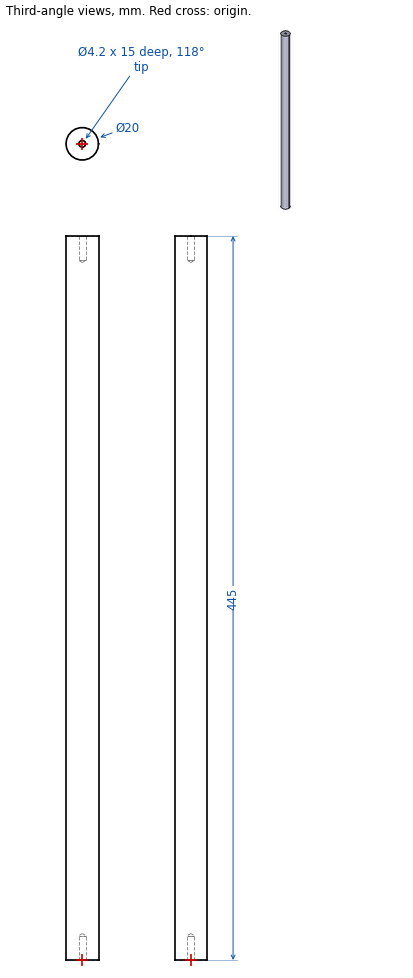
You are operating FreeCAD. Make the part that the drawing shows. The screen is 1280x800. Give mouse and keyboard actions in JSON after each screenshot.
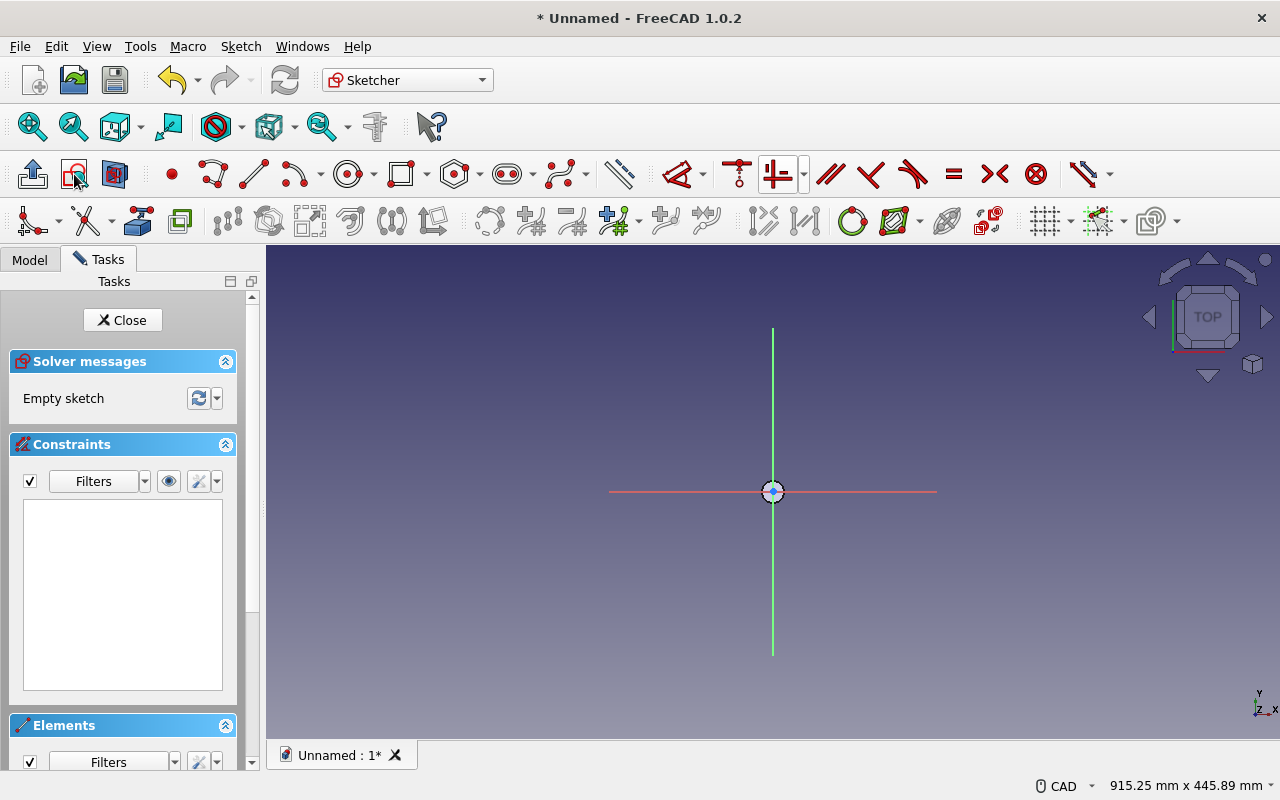
{"action": "scroll", "coordinate": [777, 492], "scroll_direction": "up", "scroll_amount": 15}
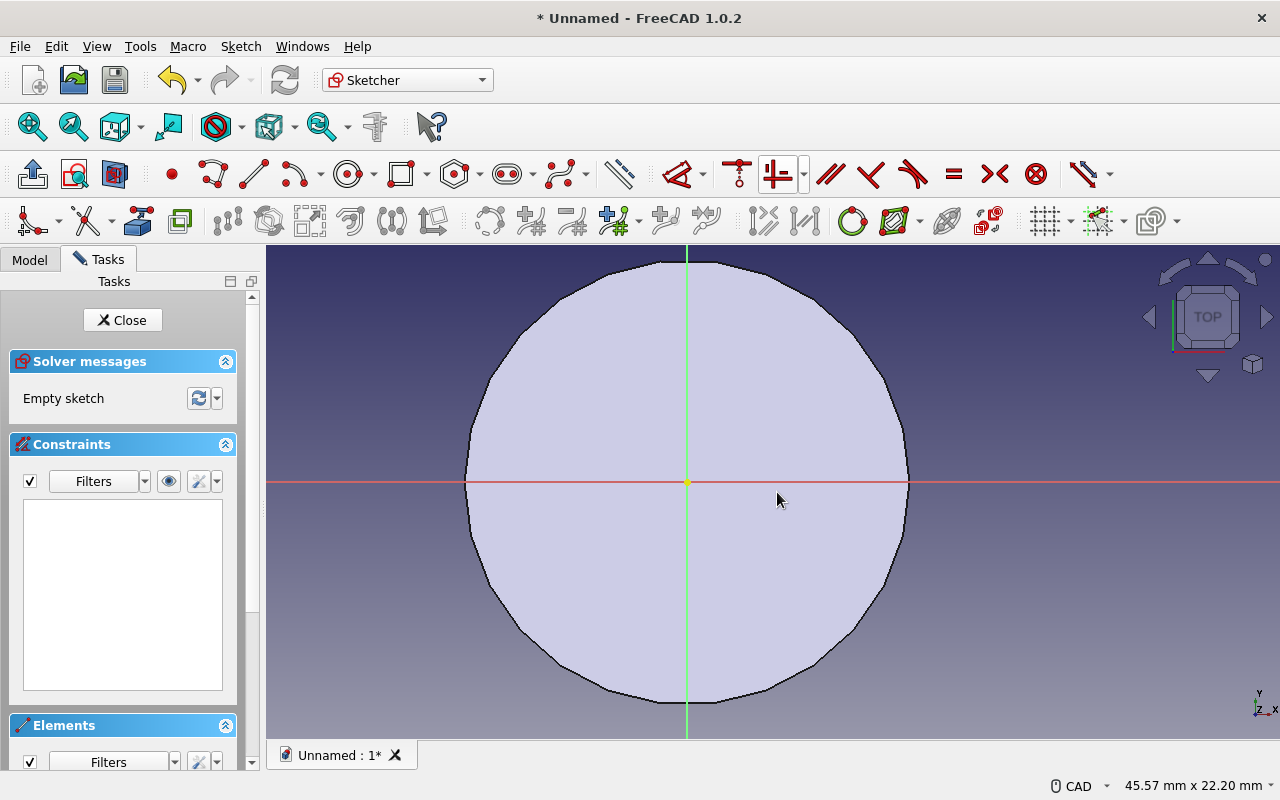
{"action": "scroll", "coordinate": [680, 478], "scroll_direction": "up", "scroll_amount": 6}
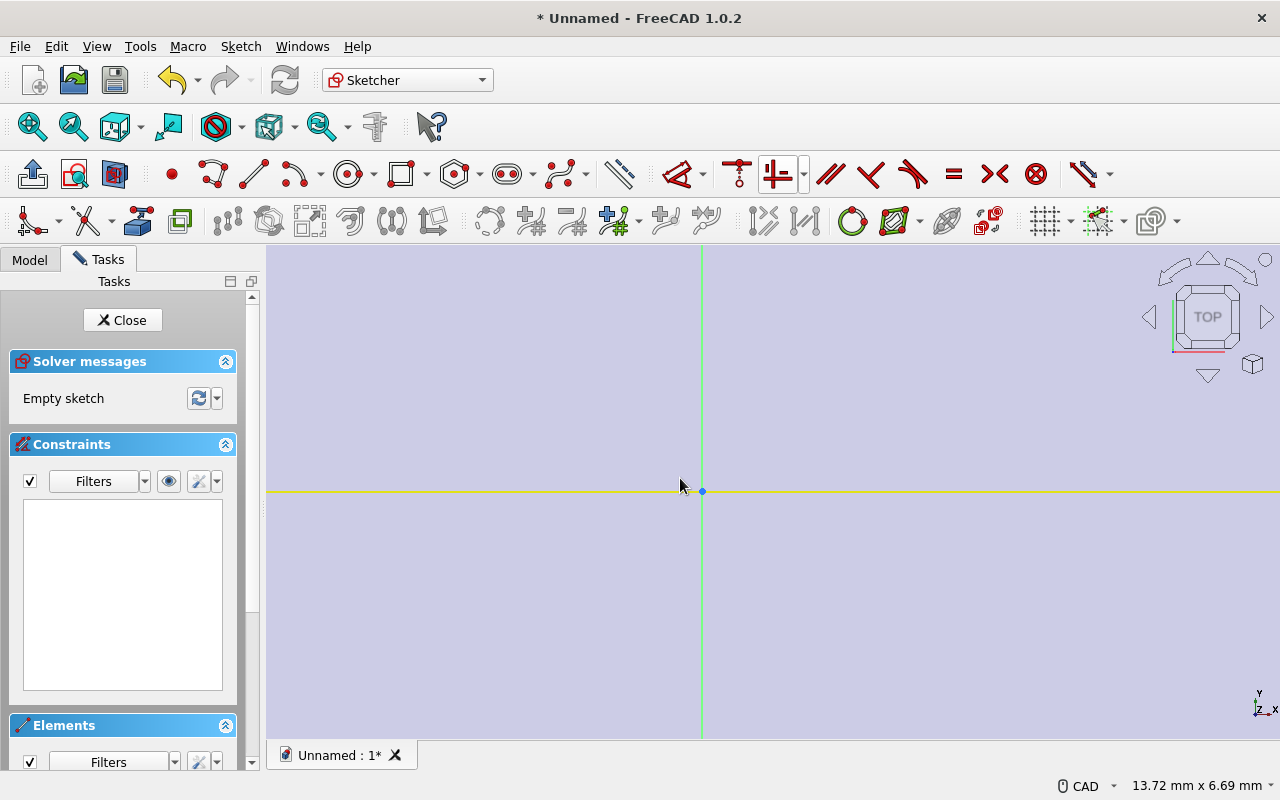
{"action": "key", "text": "g c"}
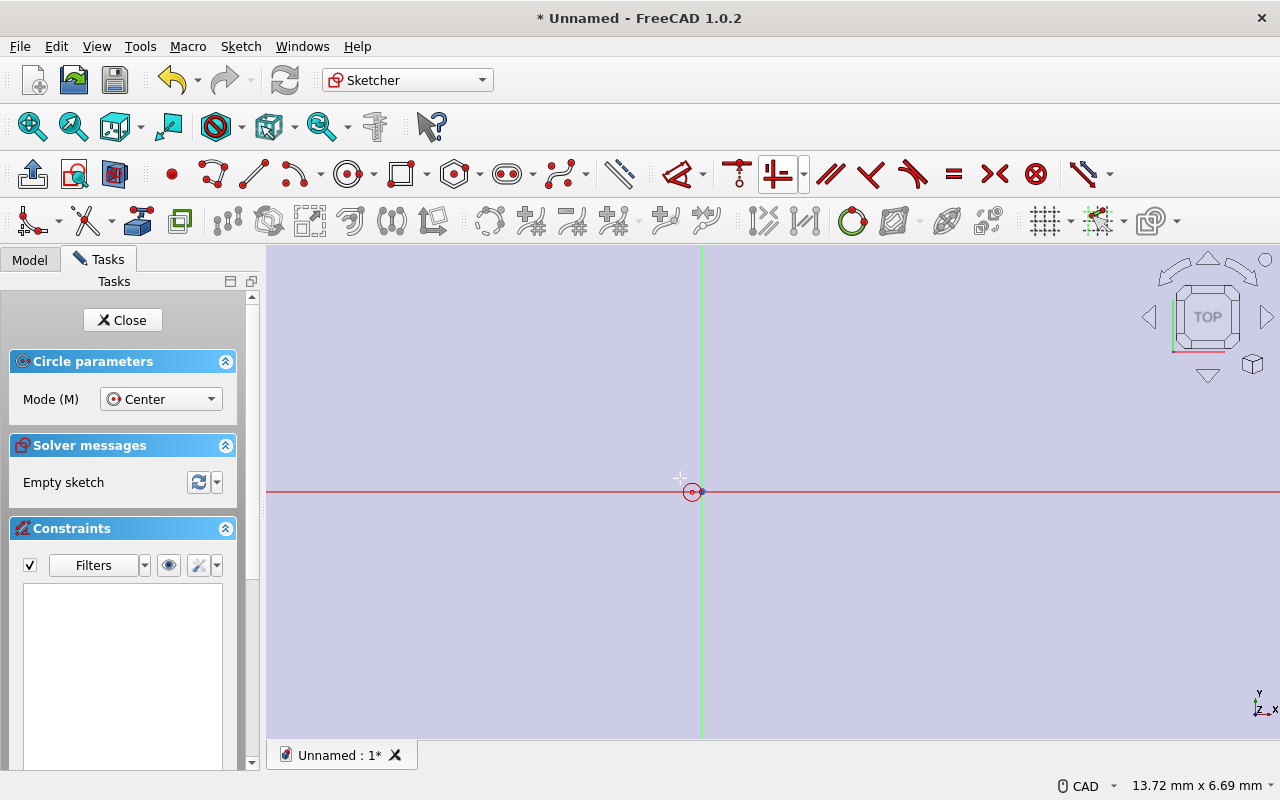
{"action": "left_click", "coordinate": [702, 492]}
{"action": "left_click", "coordinate": [812, 382]}
{"action": "key", "text": "Escape"}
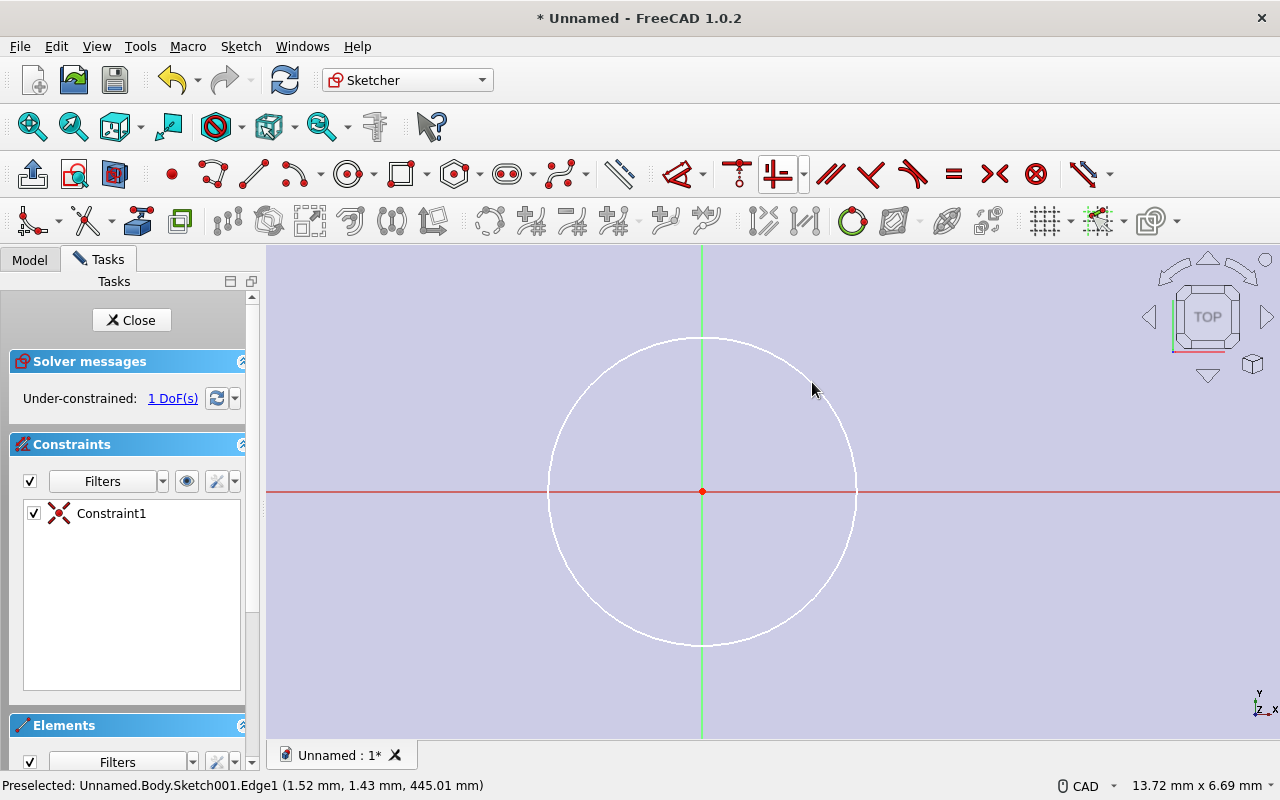
{"action": "left_click", "coordinate": [811, 382]}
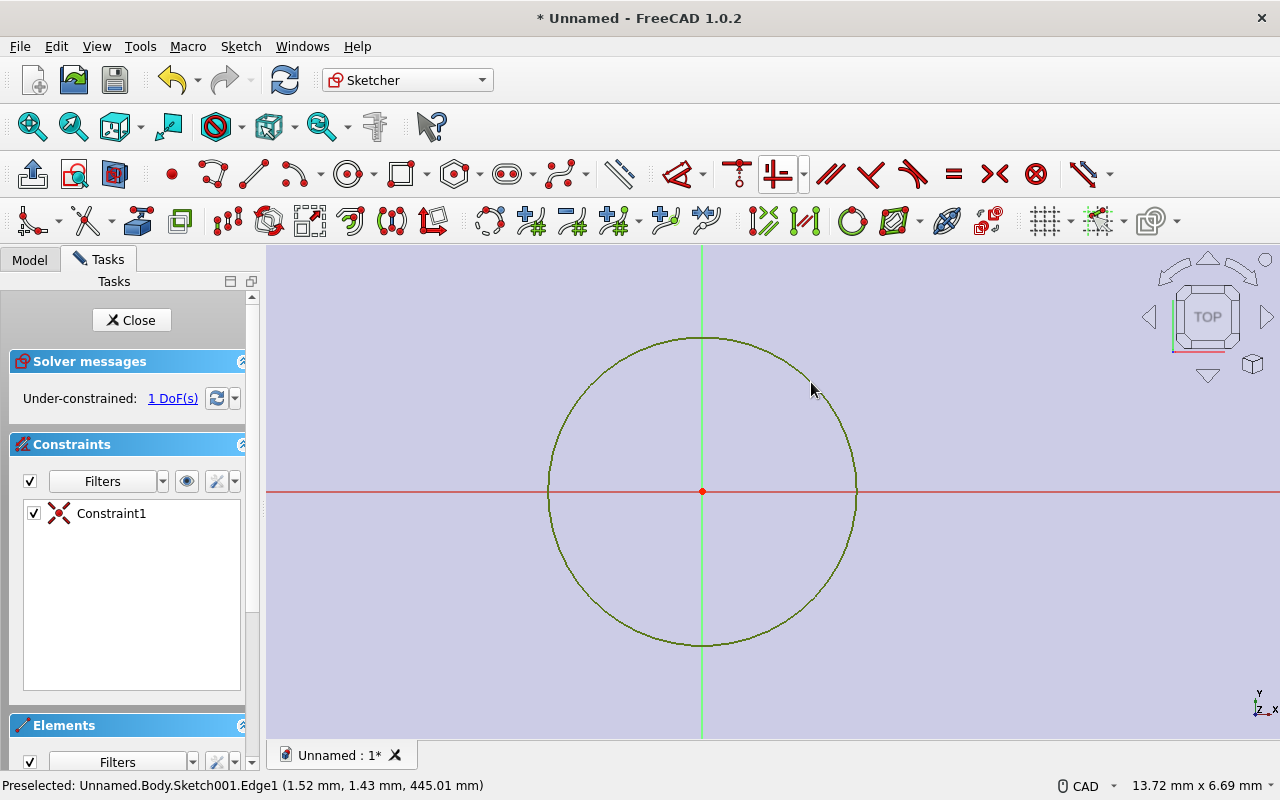
{"action": "left_click", "coordinate": [702, 174]}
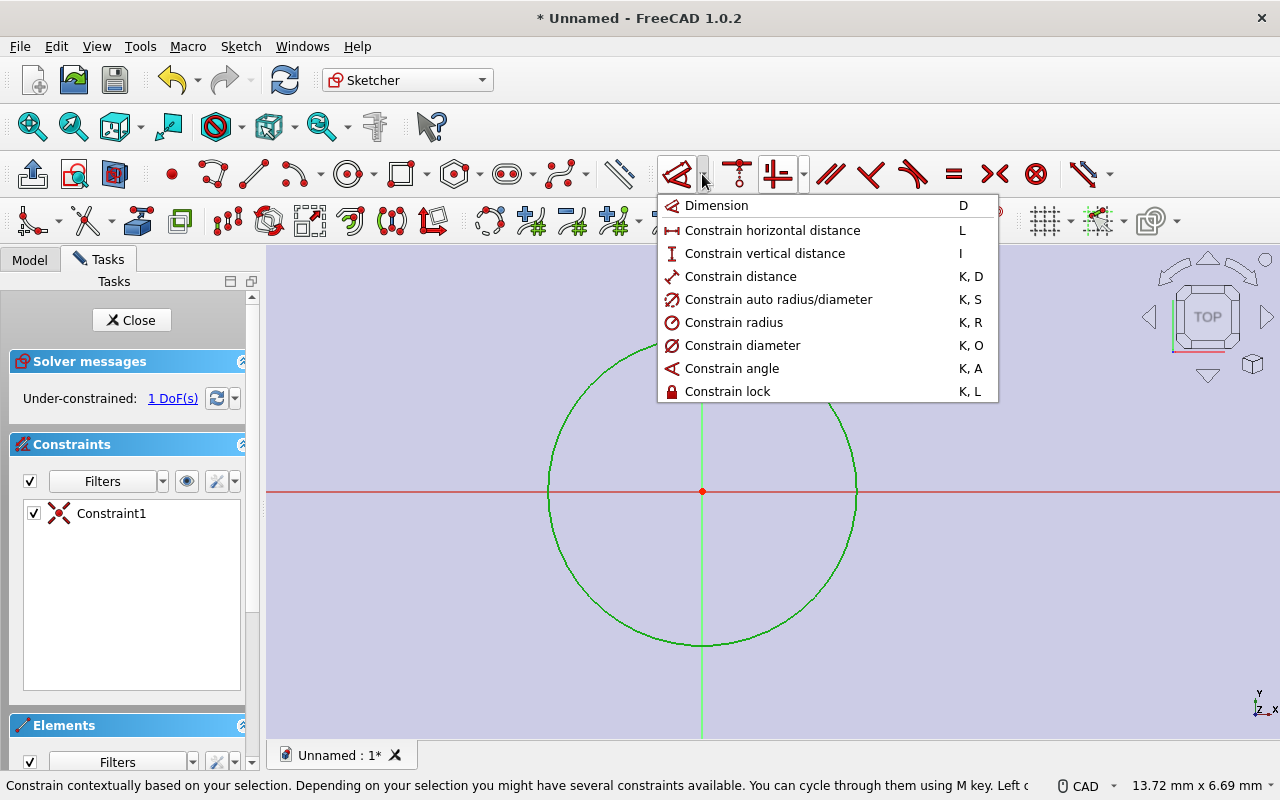
{"action": "left_click", "coordinate": [828, 346]}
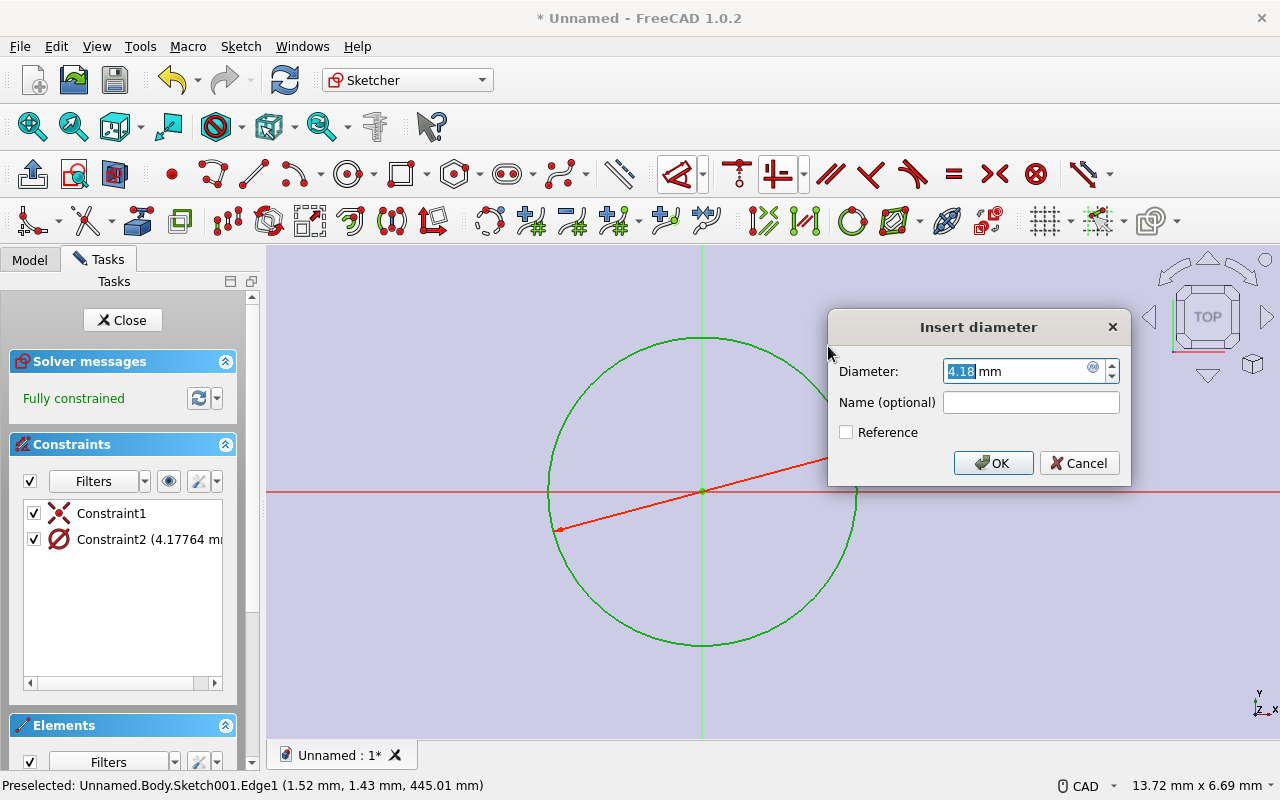
{"action": "type", "text": "4.2"}
{"action": "key", "text": "Return"}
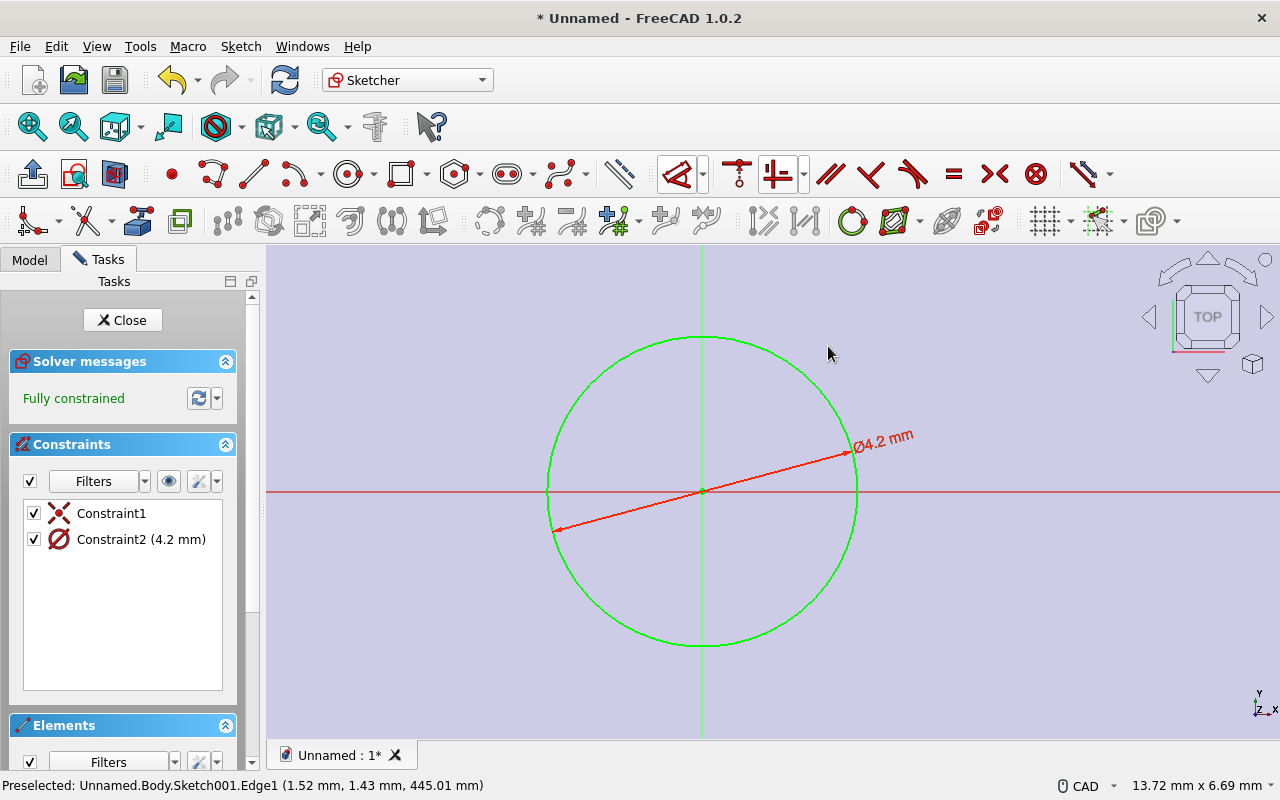
{"action": "left_click", "coordinate": [123, 320]}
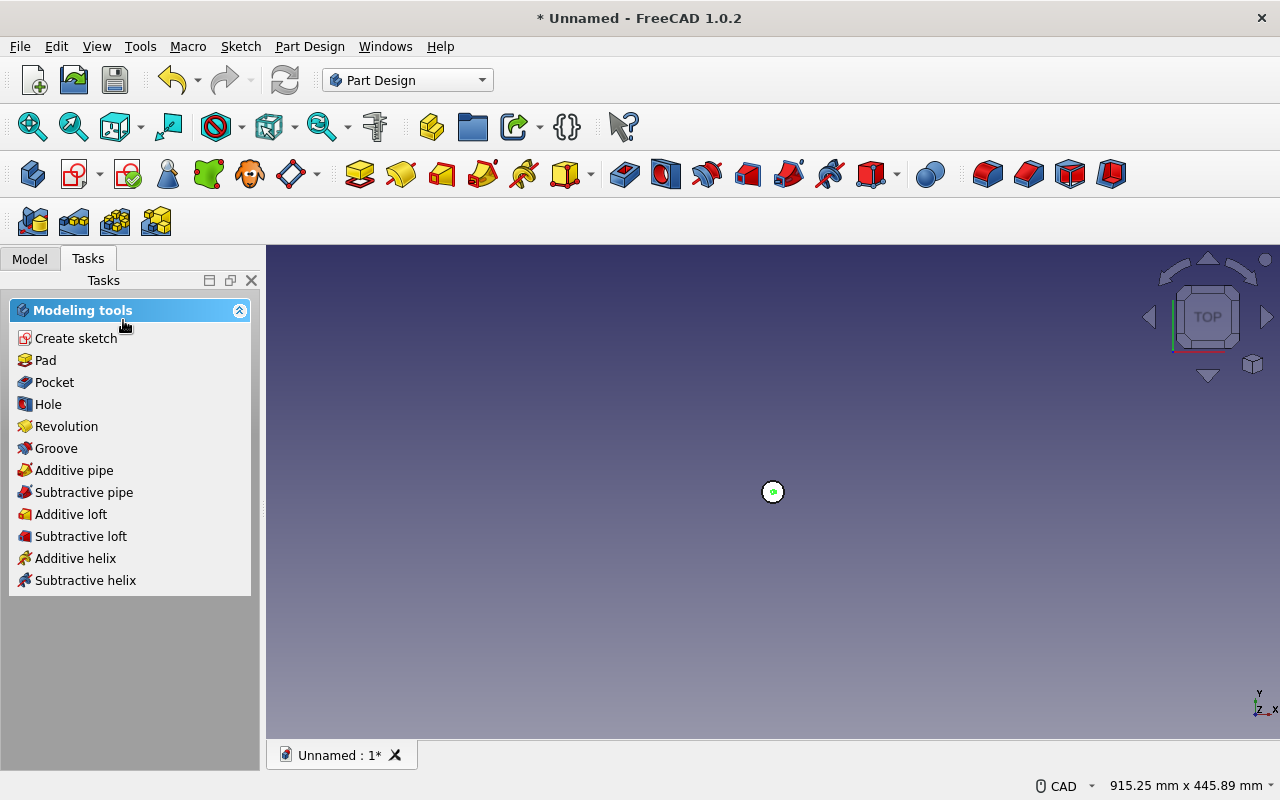
{"action": "left_click", "coordinate": [666, 174]}